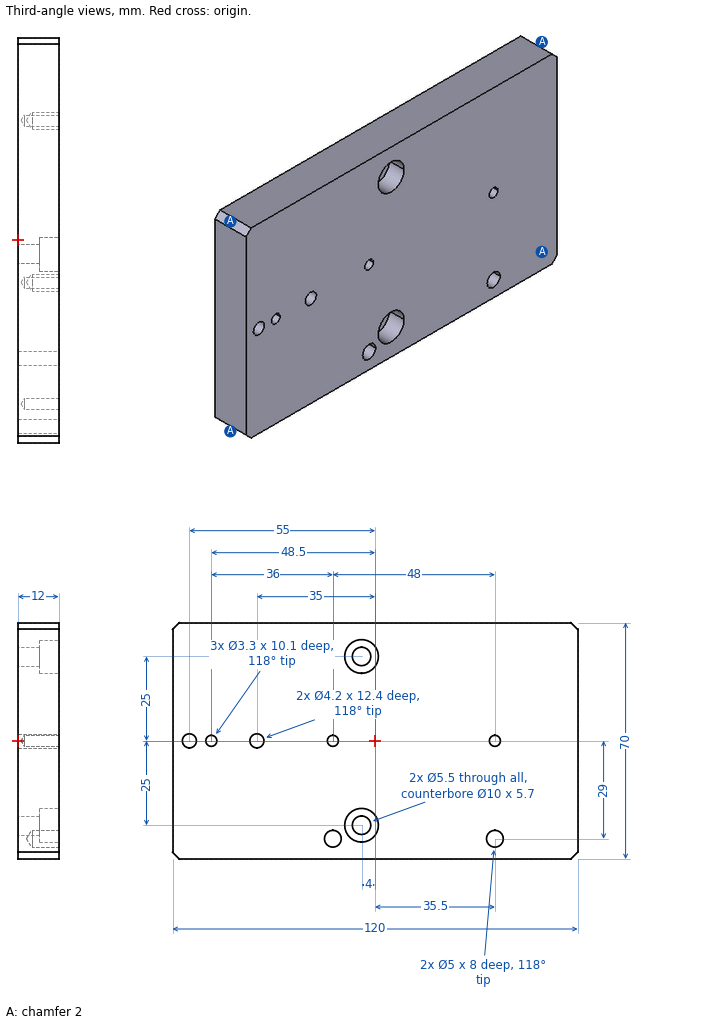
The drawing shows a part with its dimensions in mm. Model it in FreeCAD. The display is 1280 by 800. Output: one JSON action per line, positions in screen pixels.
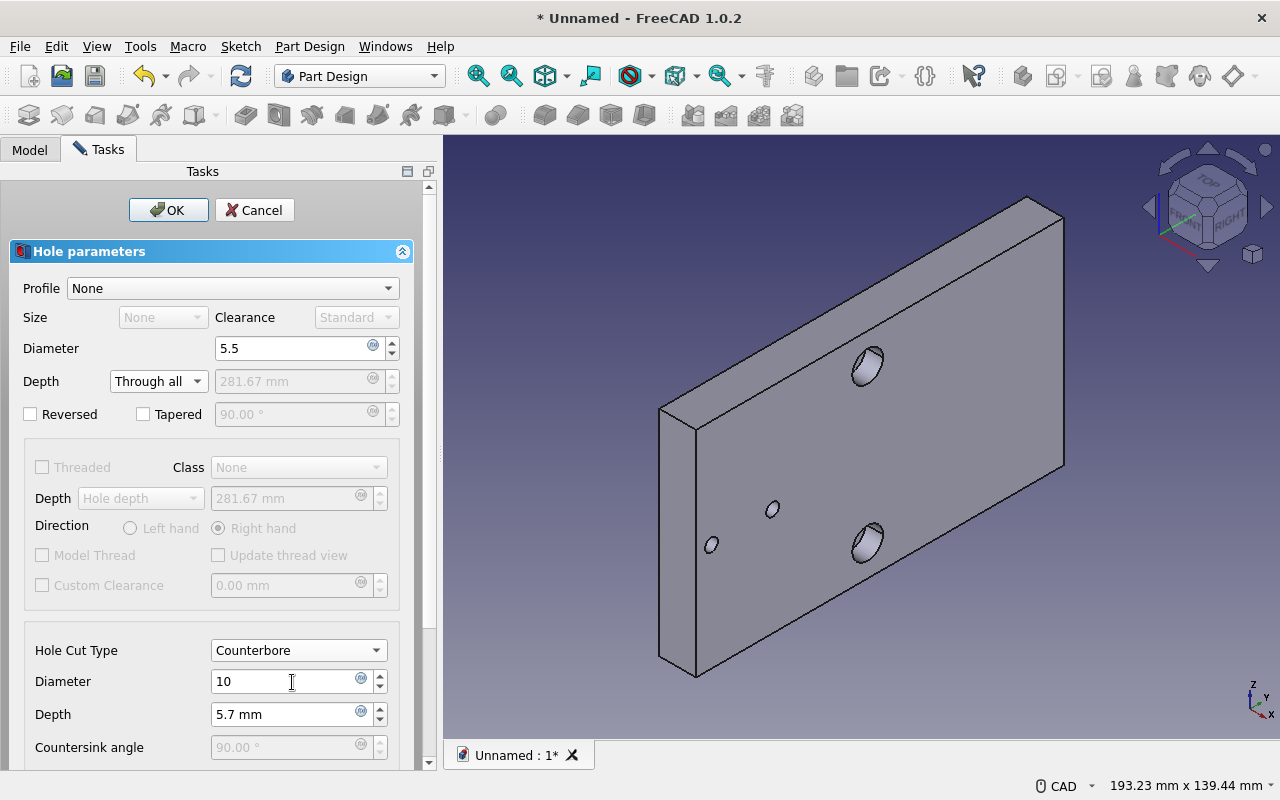
{"action": "left_click", "coordinate": [169, 210]}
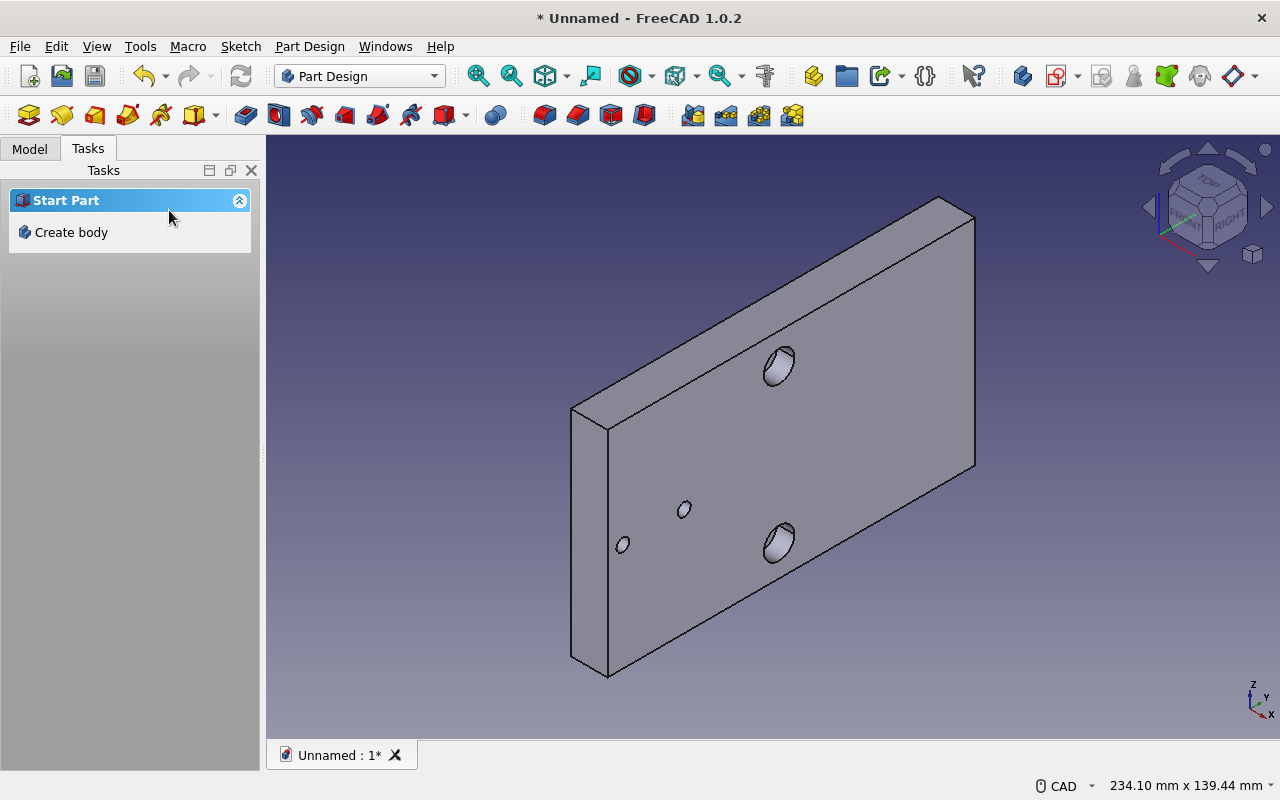
{"action": "left_click", "coordinate": [844, 416]}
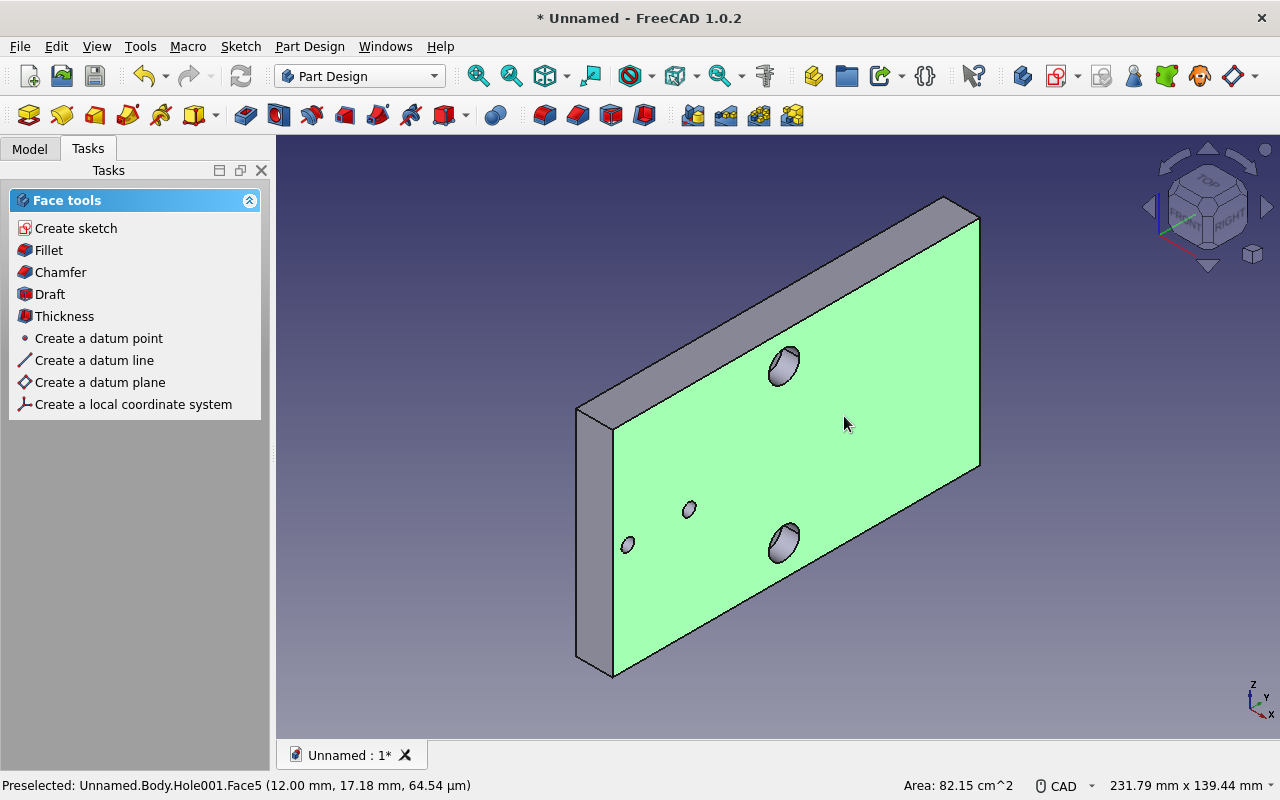
{"action": "left_click", "coordinate": [1056, 76]}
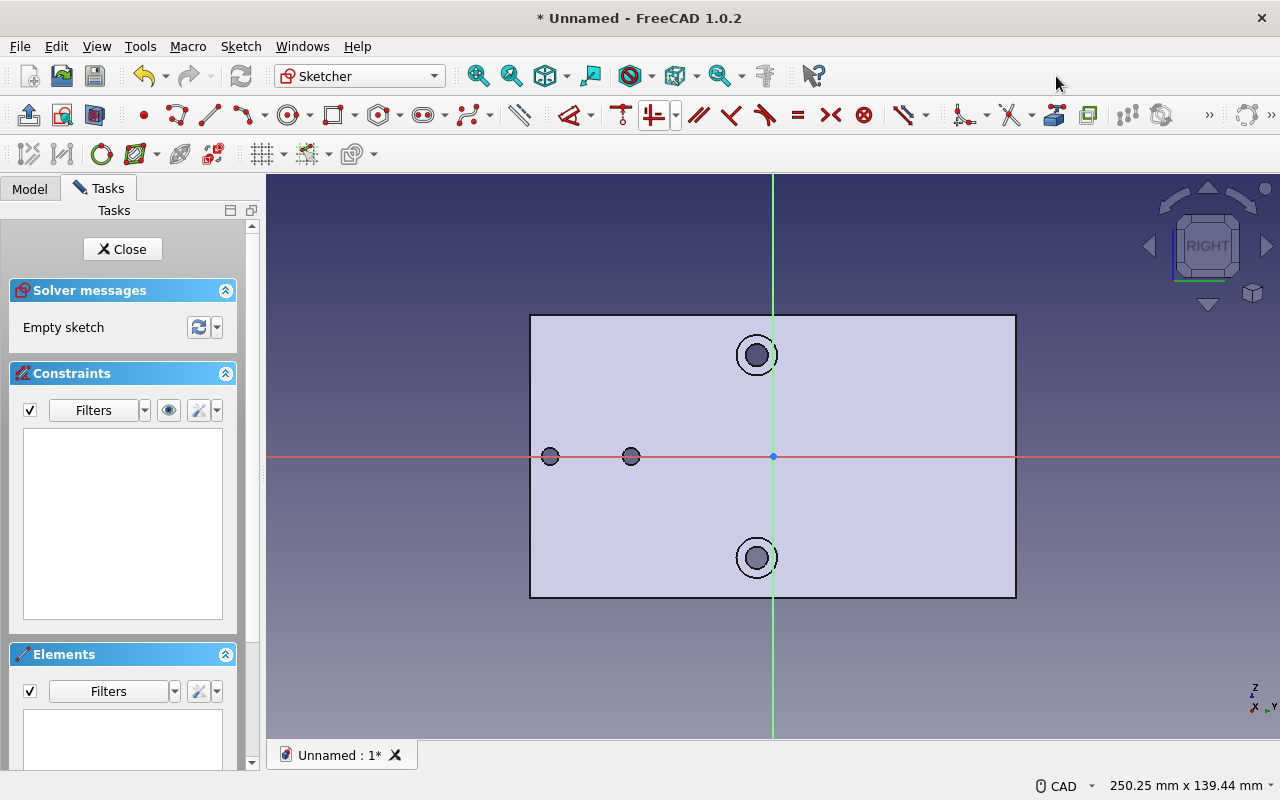
{"action": "scroll", "coordinate": [832, 457], "scroll_direction": "up", "scroll_amount": 2}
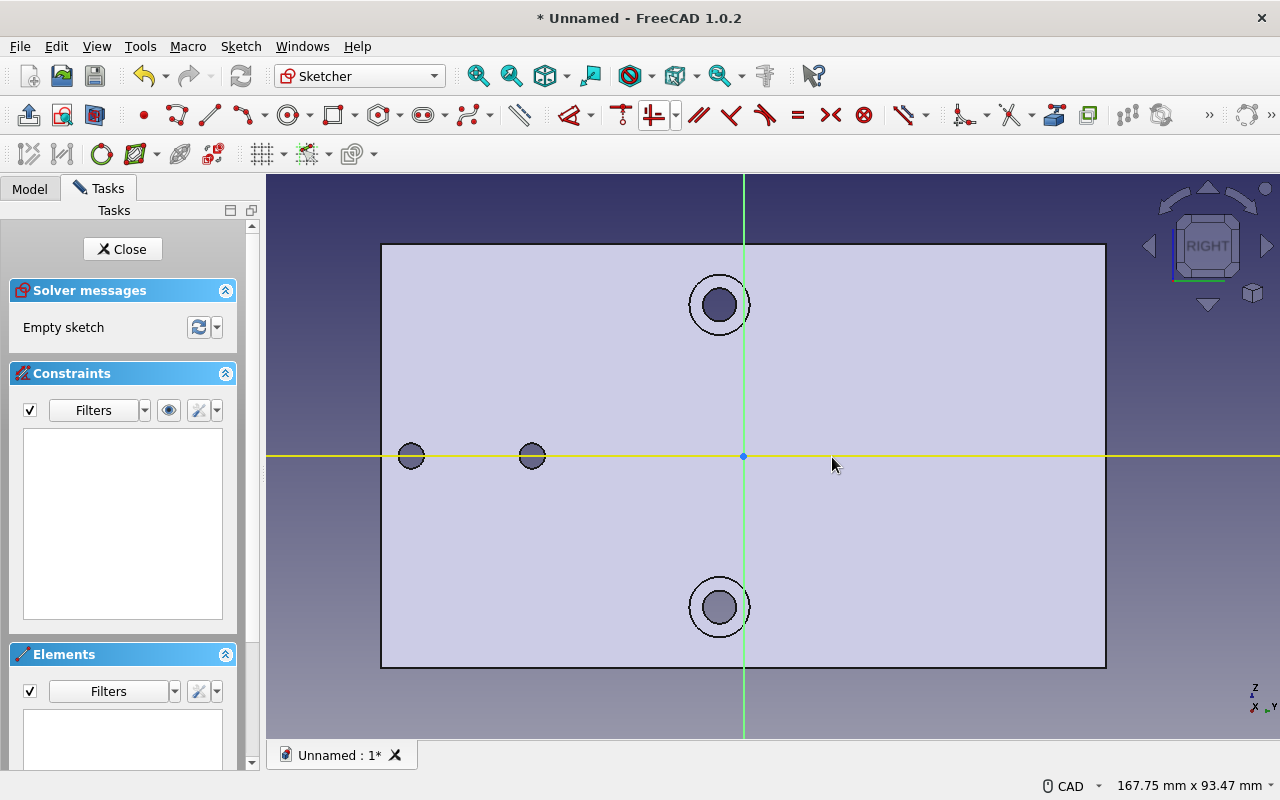
{"action": "left_click", "coordinate": [288, 116]}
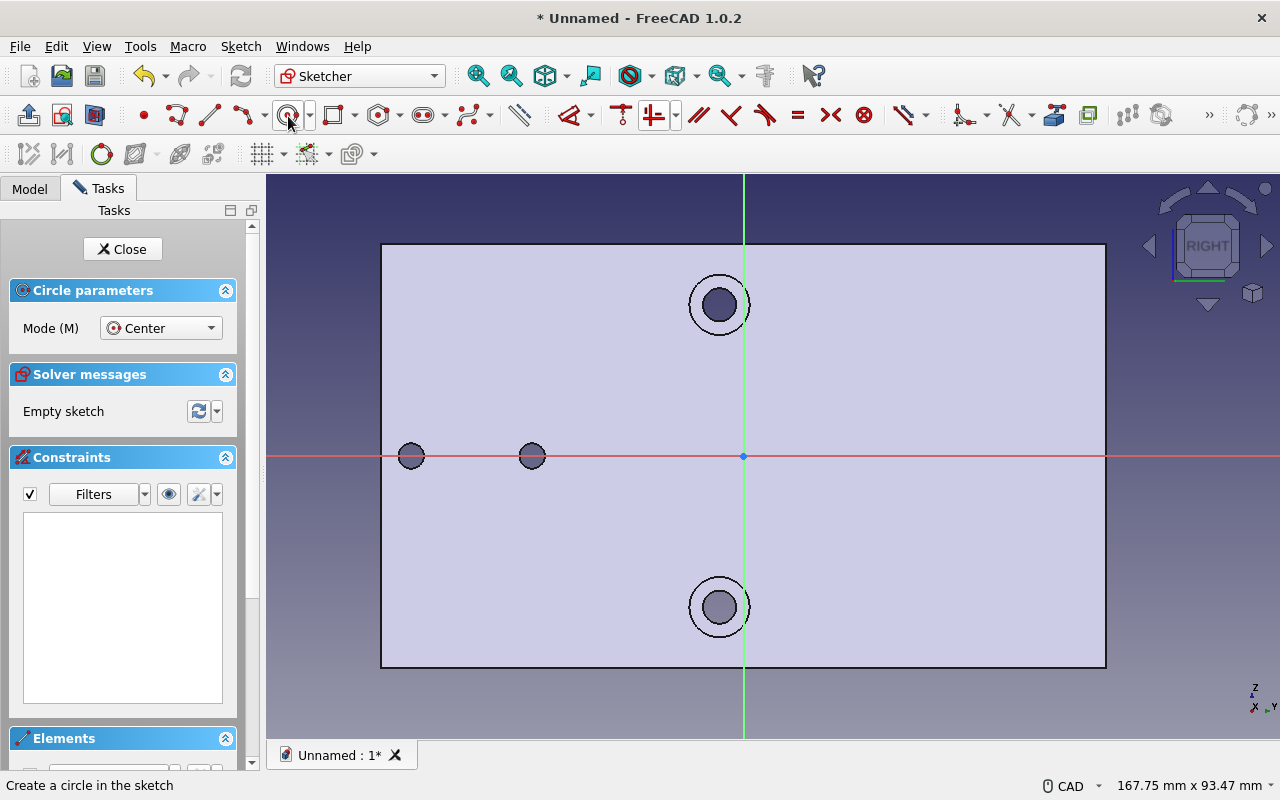
{"action": "scroll", "coordinate": [451, 456], "scroll_direction": "up", "scroll_amount": 5}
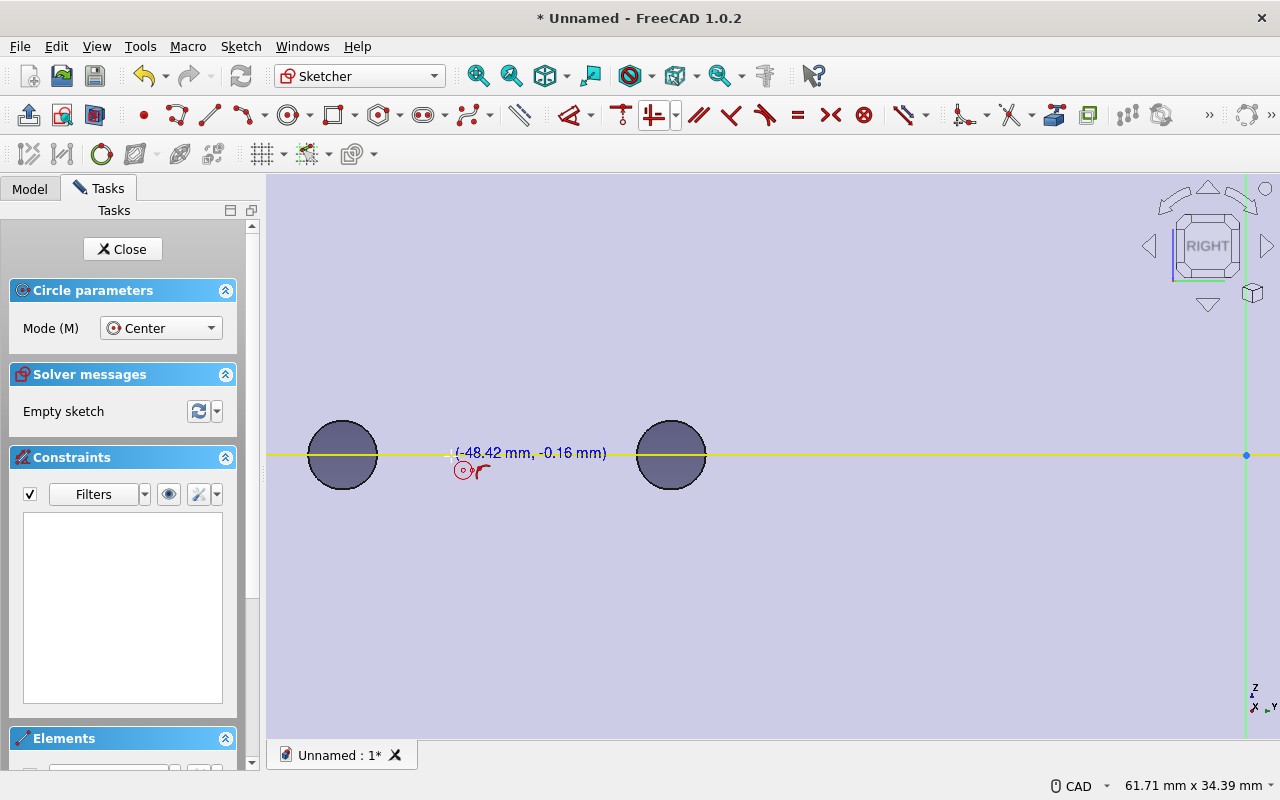
{"action": "left_click", "coordinate": [449, 455]}
{"action": "left_click", "coordinate": [469, 436]}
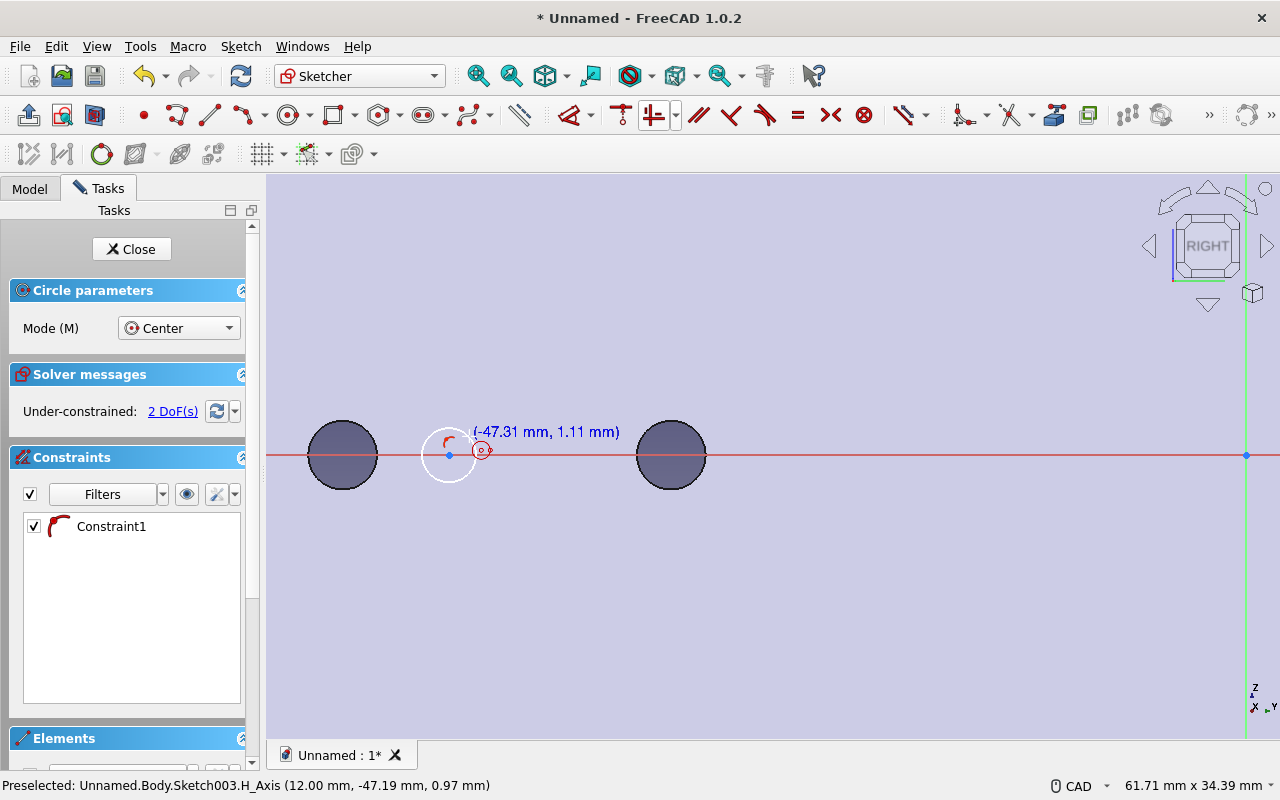
{"action": "left_click", "coordinate": [1041, 455]}
{"action": "left_click", "coordinate": [1060, 436]}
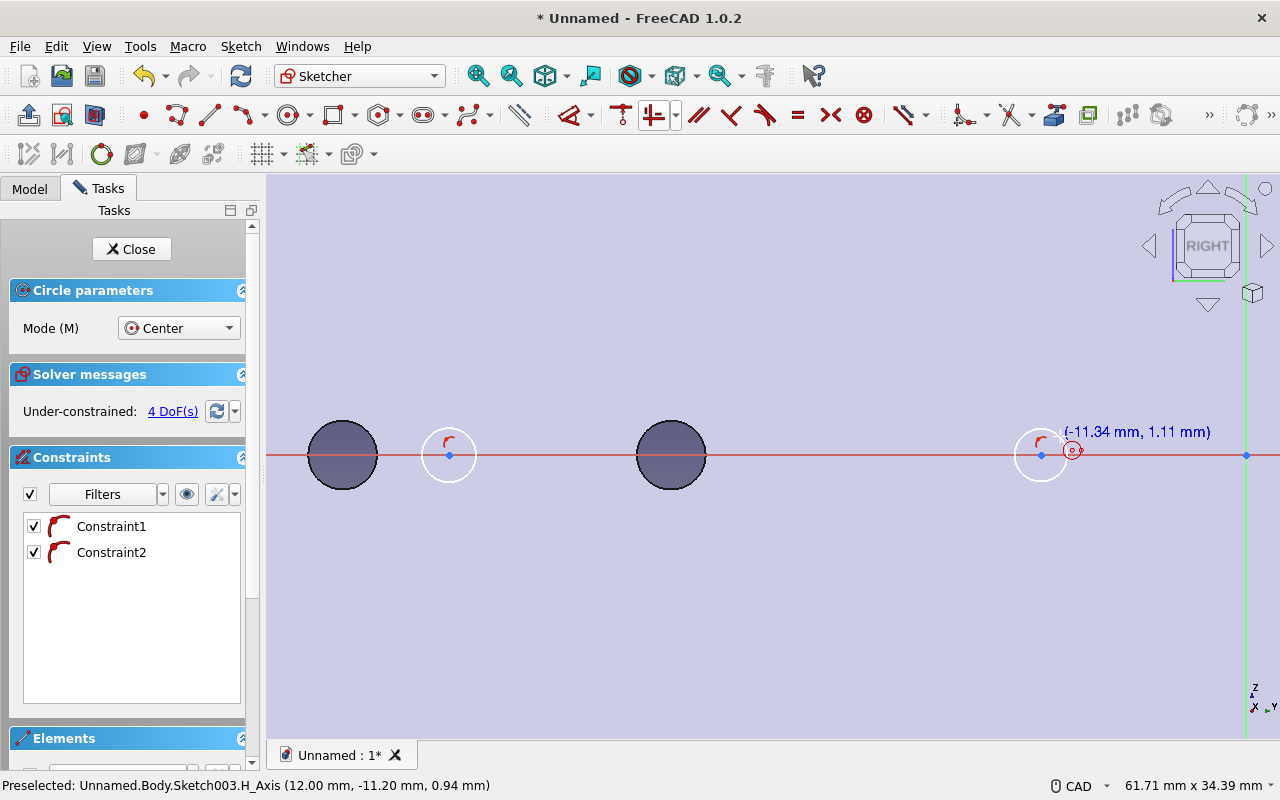
{"action": "scroll", "coordinate": [451, 457], "scroll_direction": "down", "scroll_amount": 5}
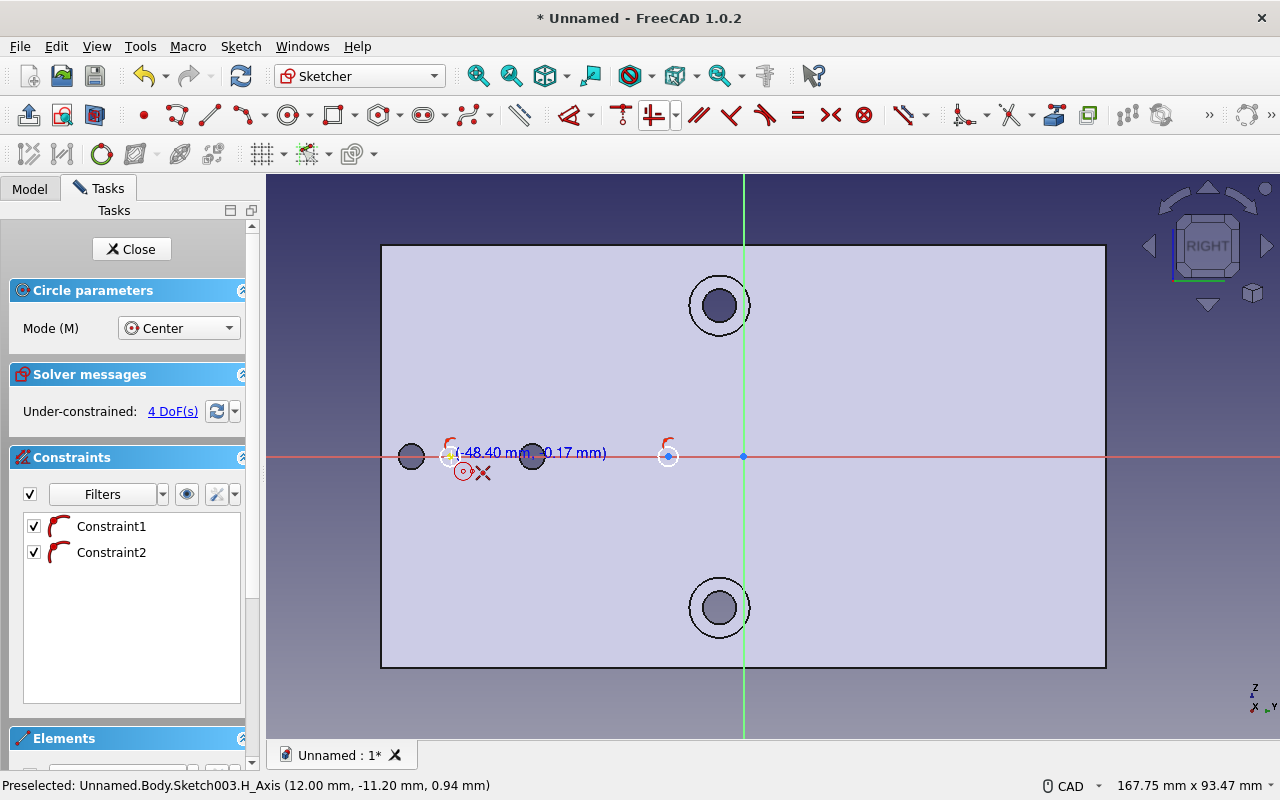
{"action": "scroll", "coordinate": [958, 457], "scroll_direction": "up", "scroll_amount": 5}